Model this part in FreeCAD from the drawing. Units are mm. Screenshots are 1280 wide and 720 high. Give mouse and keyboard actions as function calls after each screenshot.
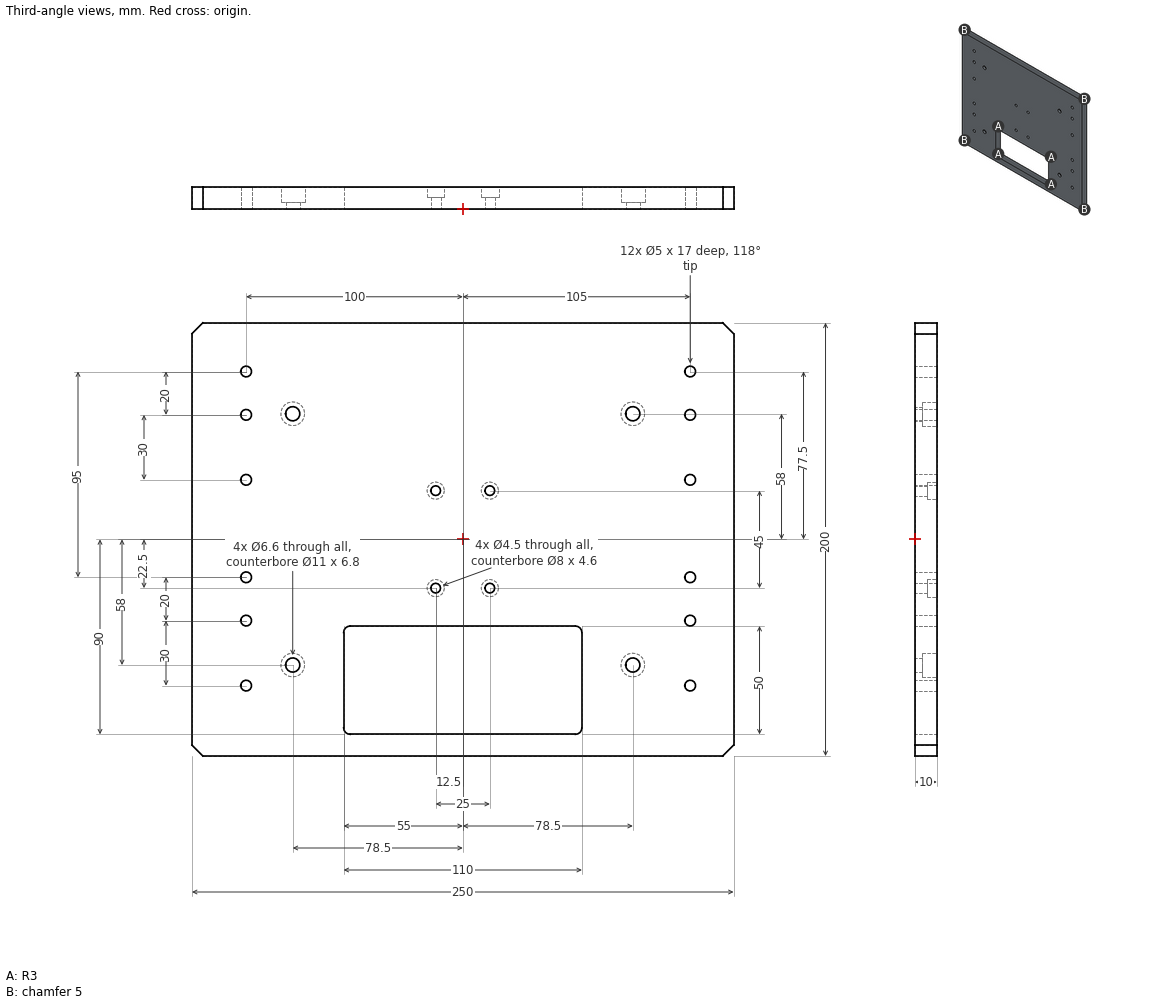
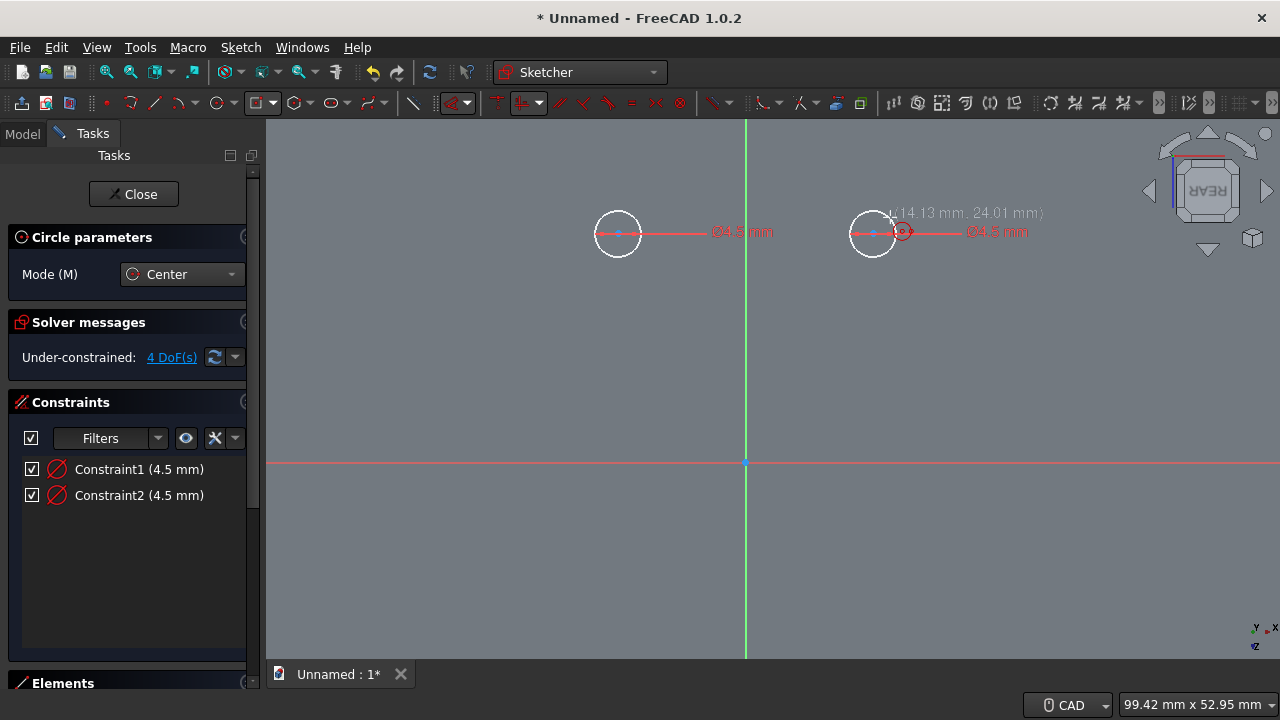
scroll(620, 239, down, 2)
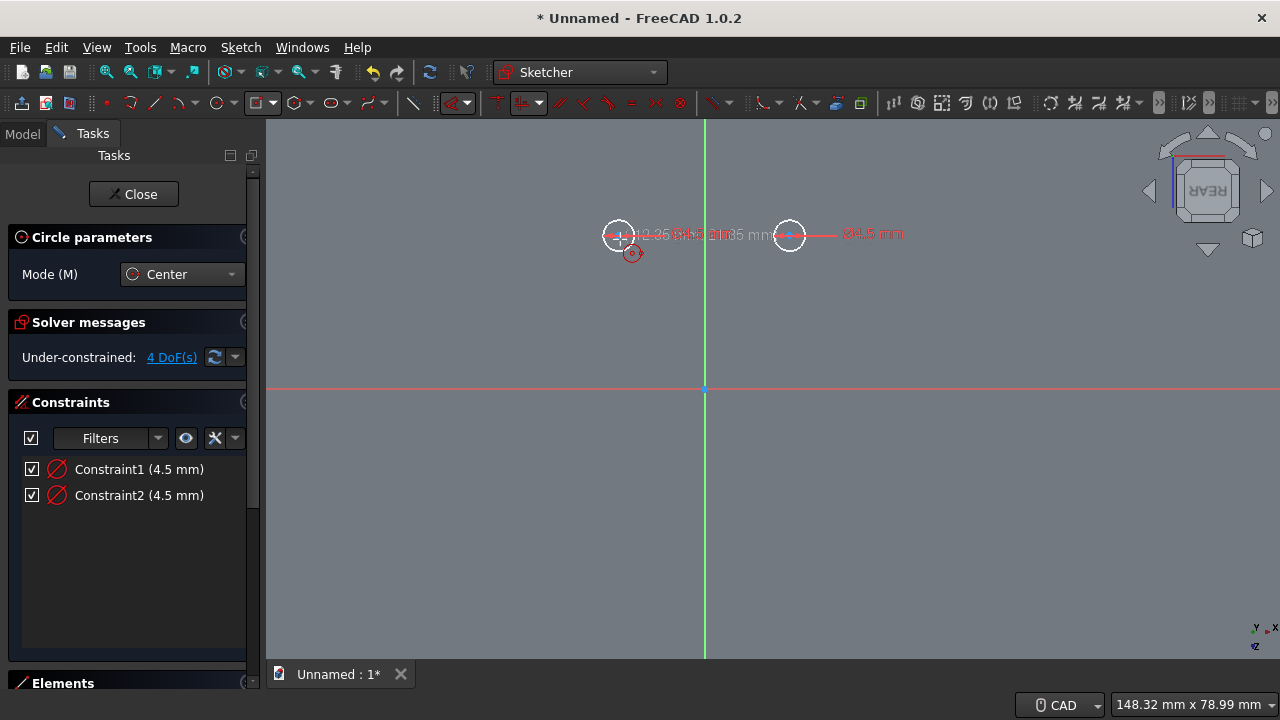
scroll(790, 543, up, 2)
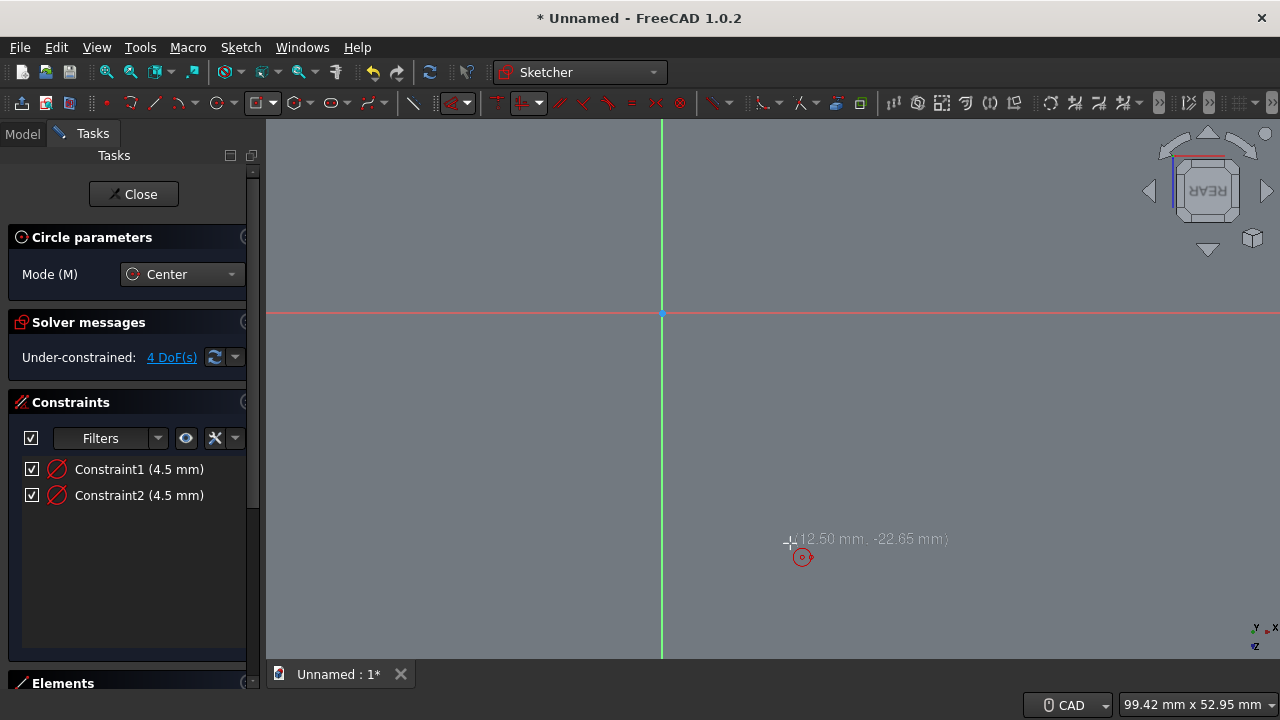
click(790, 543)
move(806, 526)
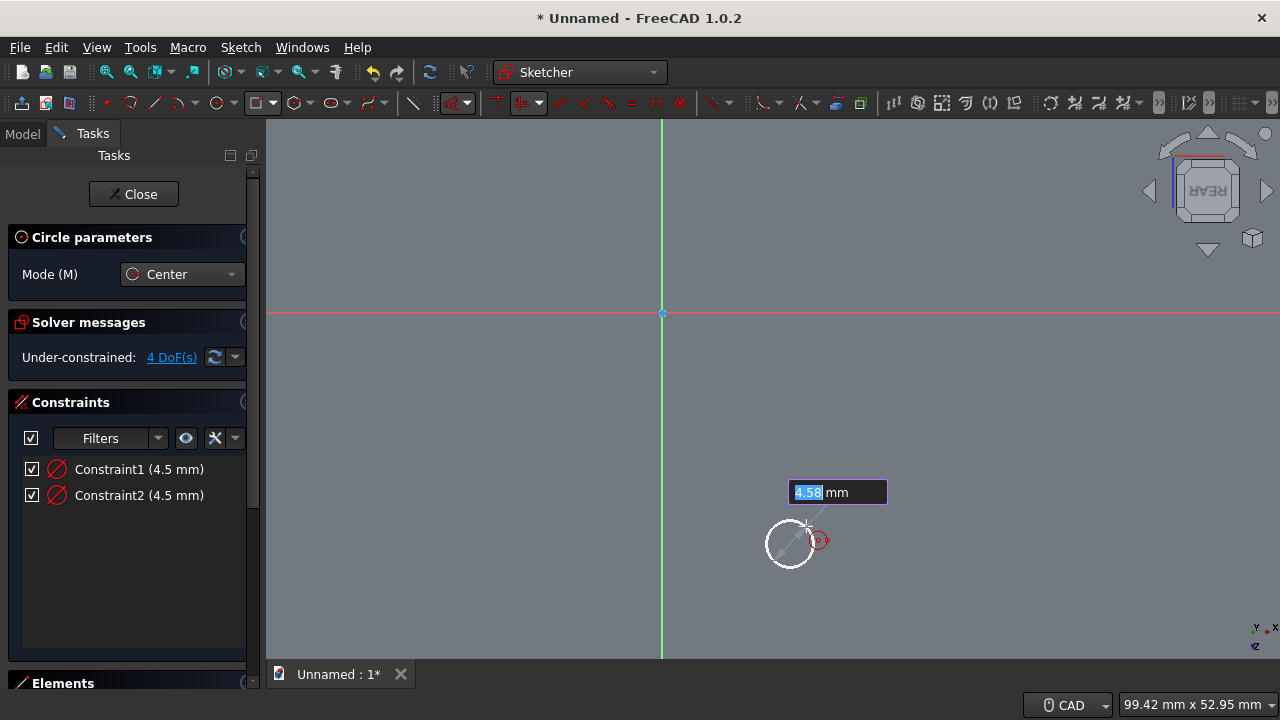
text(4.5)
key(Return)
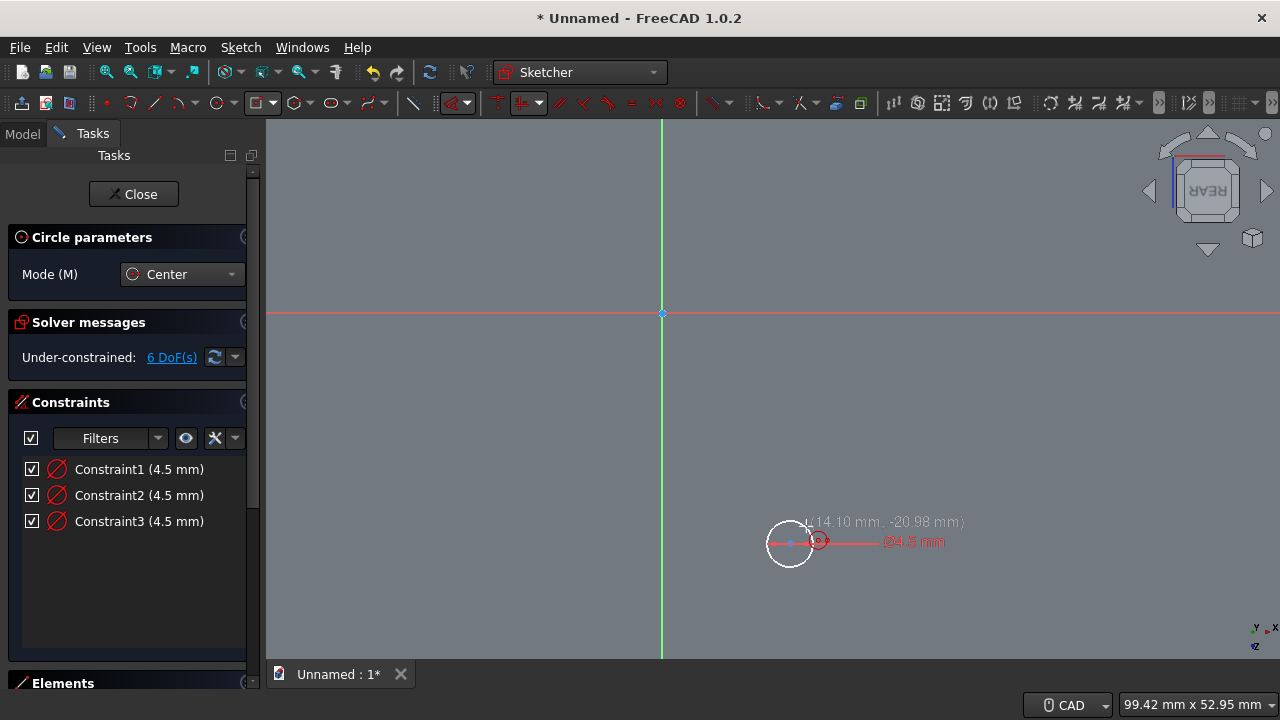
click(535, 543)
move(551, 526)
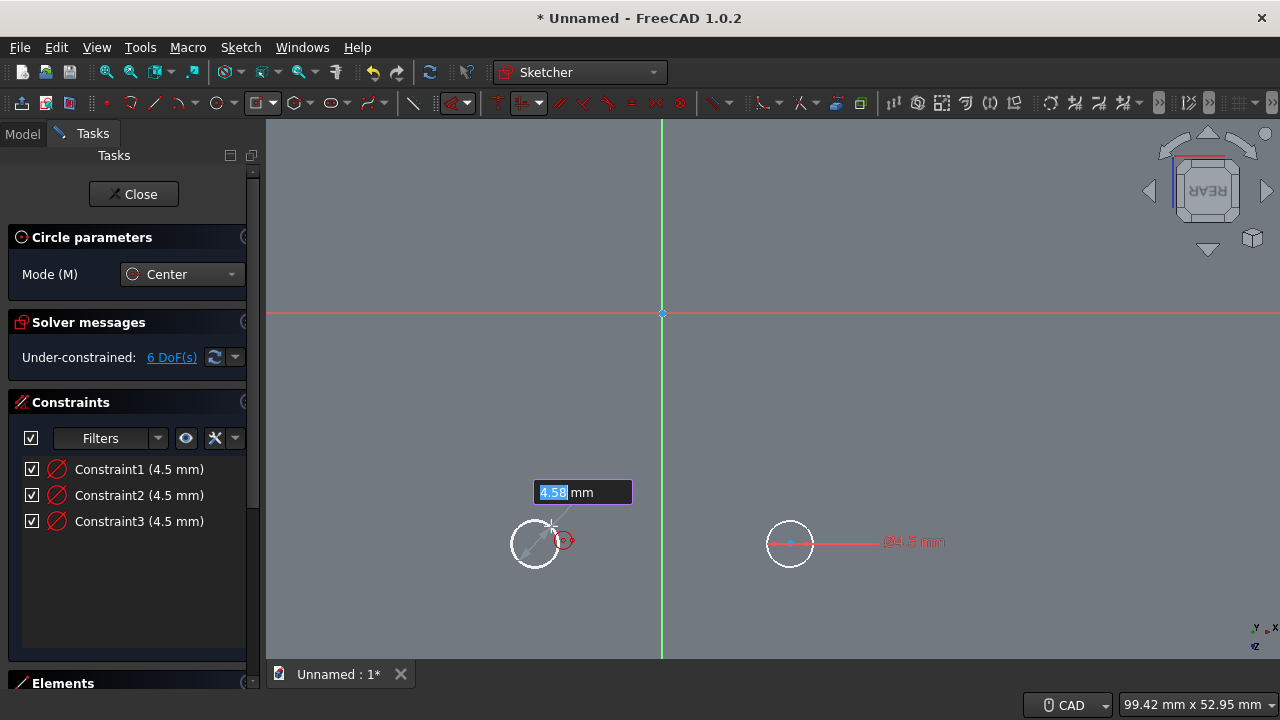
text(4.5)
key(Return)
key(Escape)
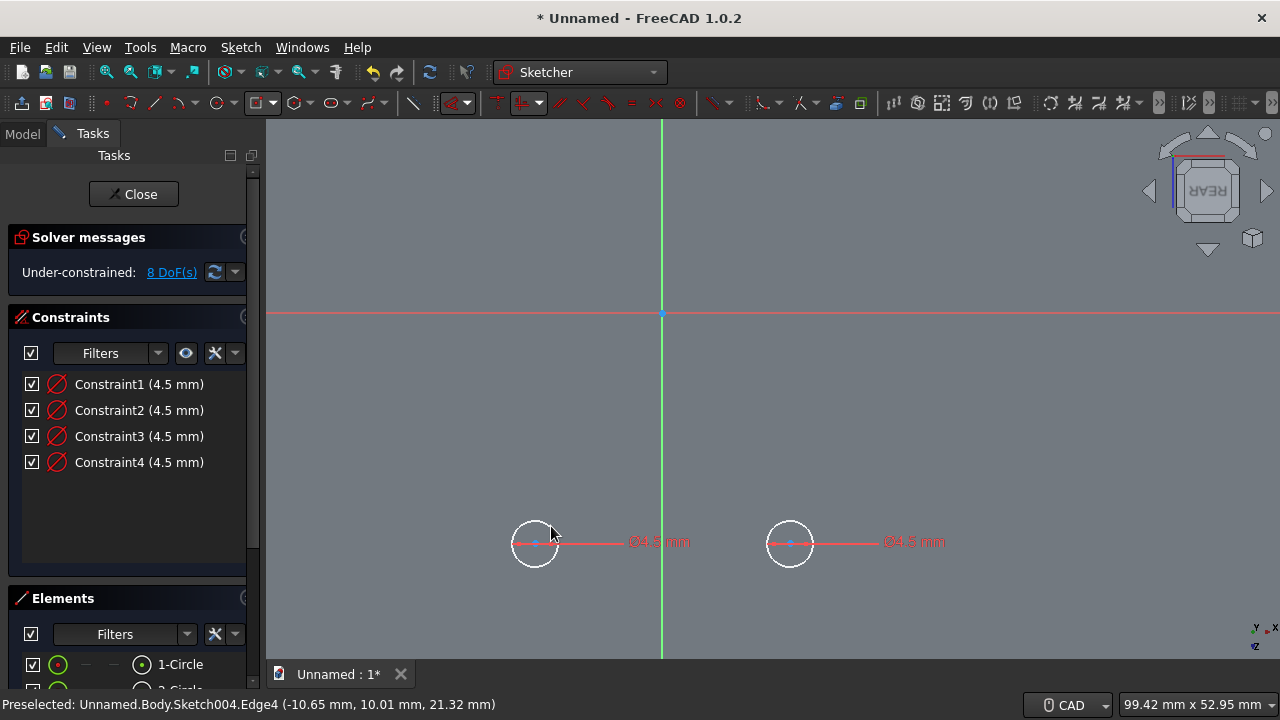
scroll(790, 543, down, 2)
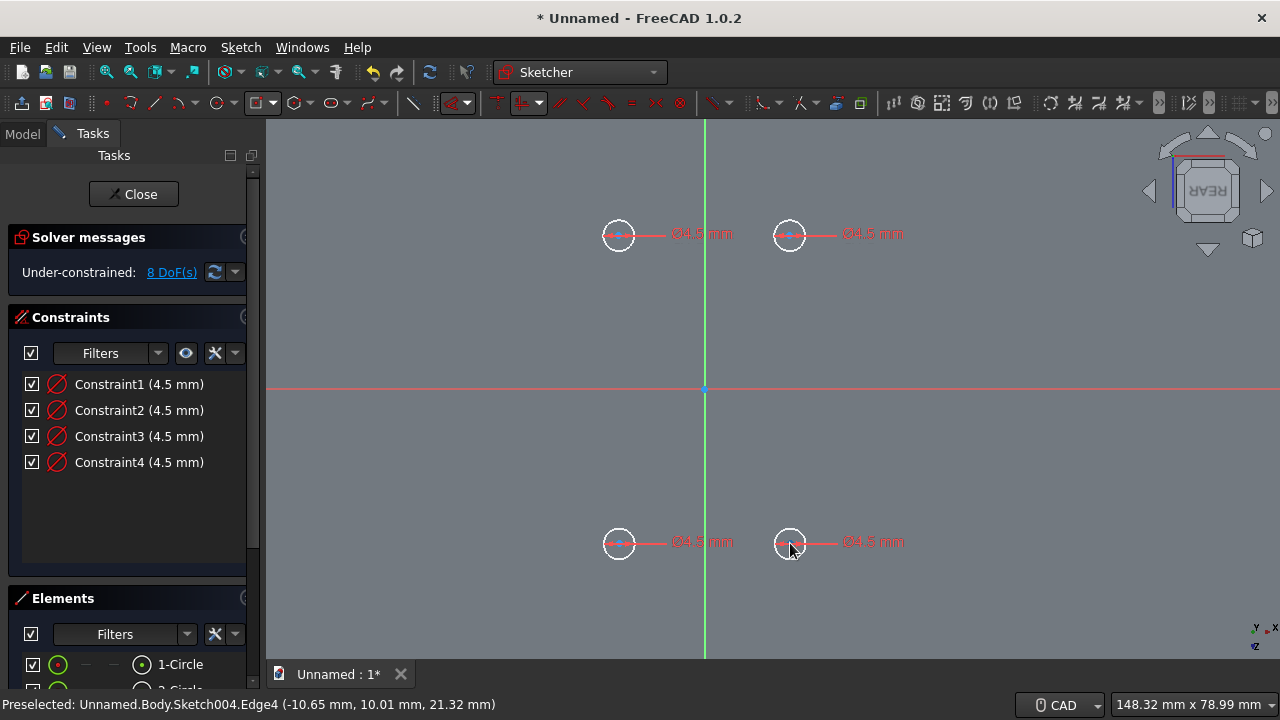
click(619, 236)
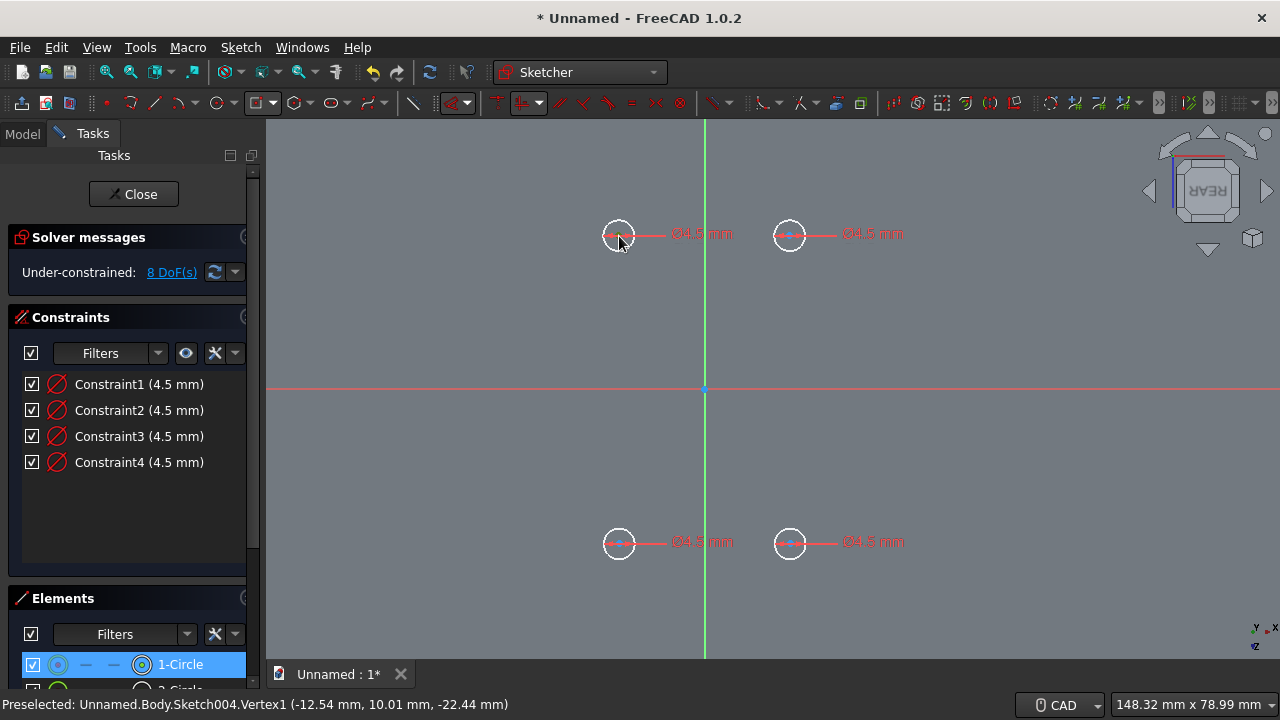
click(790, 236)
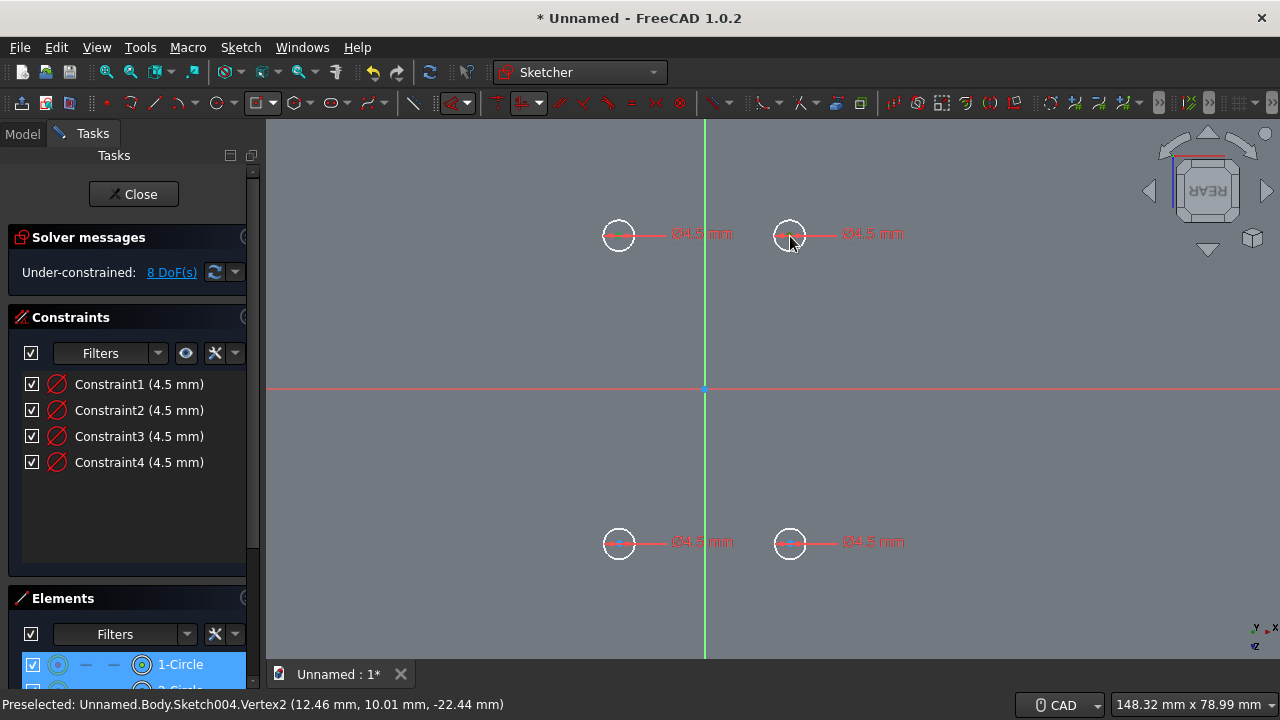
click(542, 104)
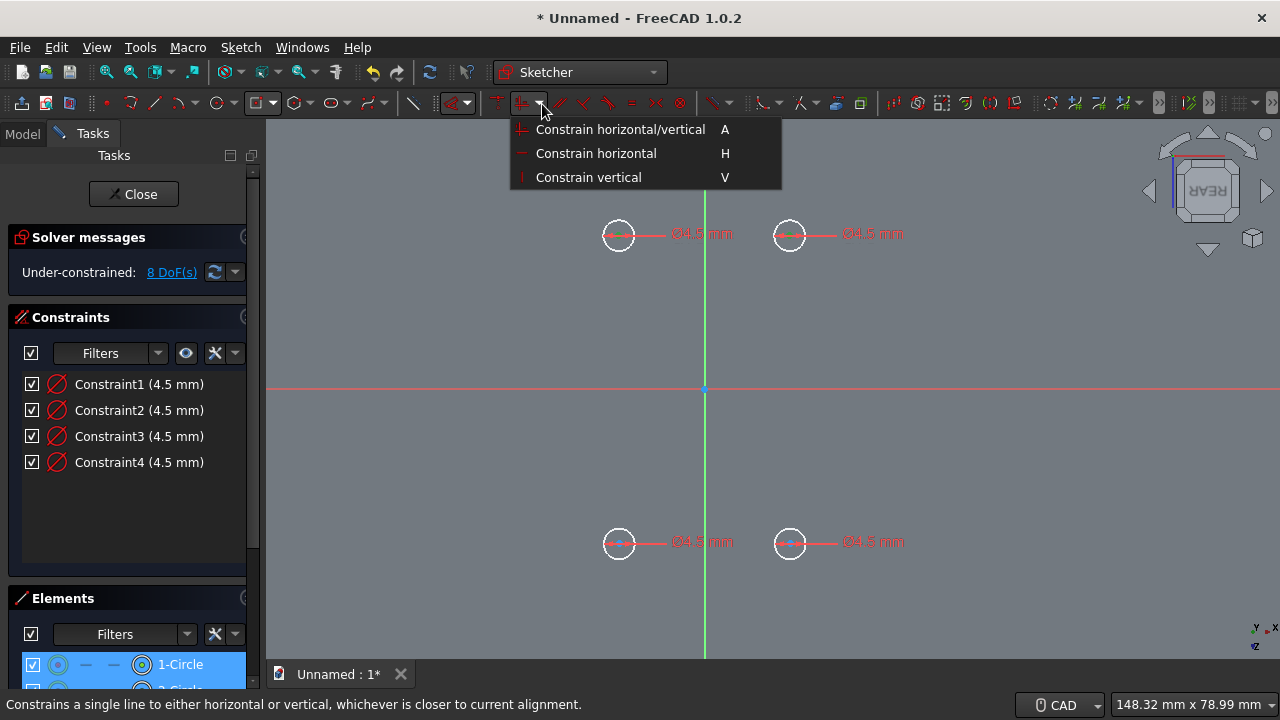
click(646, 153)